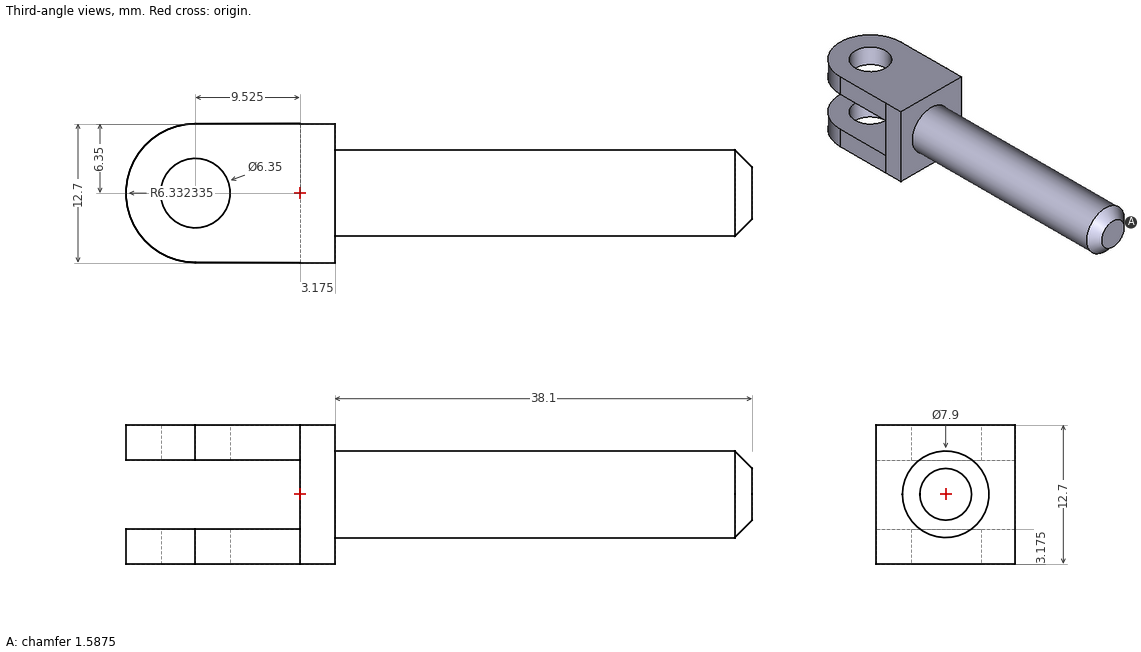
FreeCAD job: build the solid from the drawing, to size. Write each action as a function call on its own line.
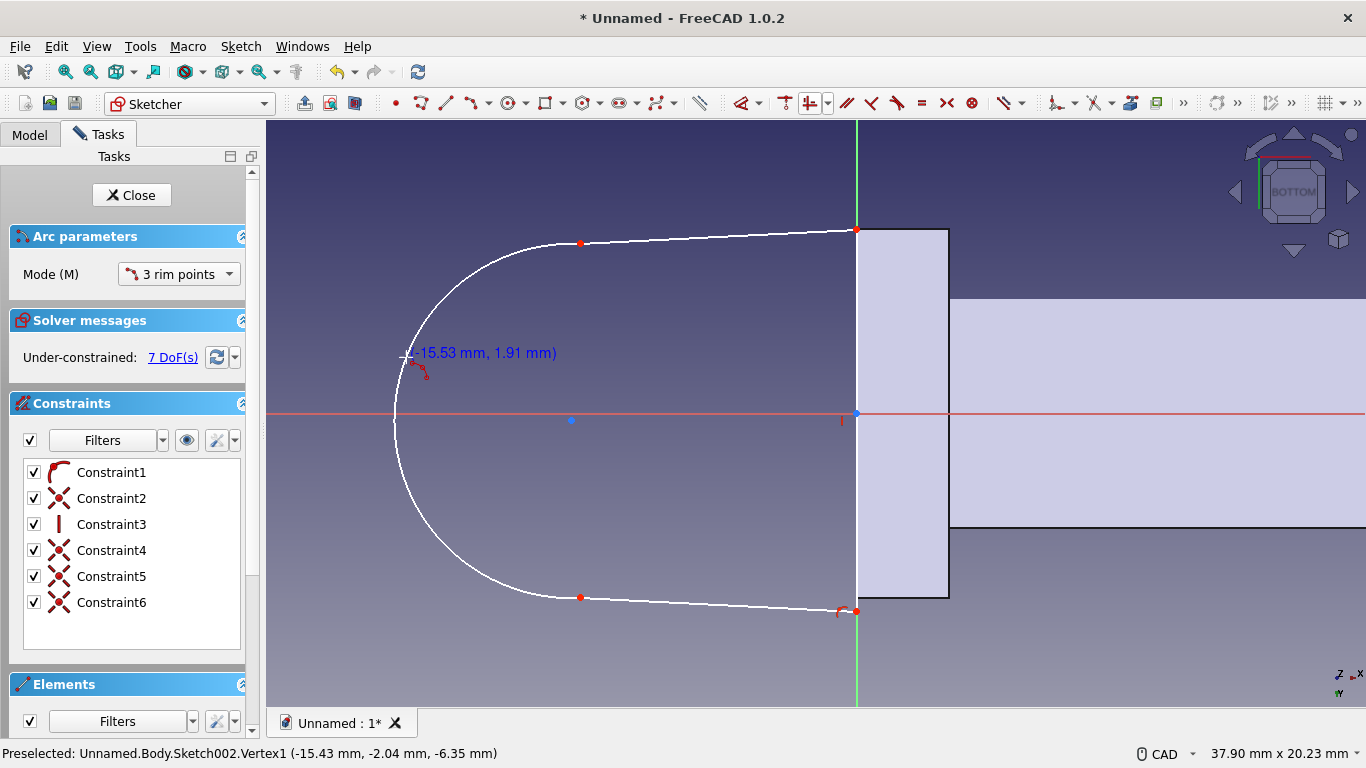
click(508, 104)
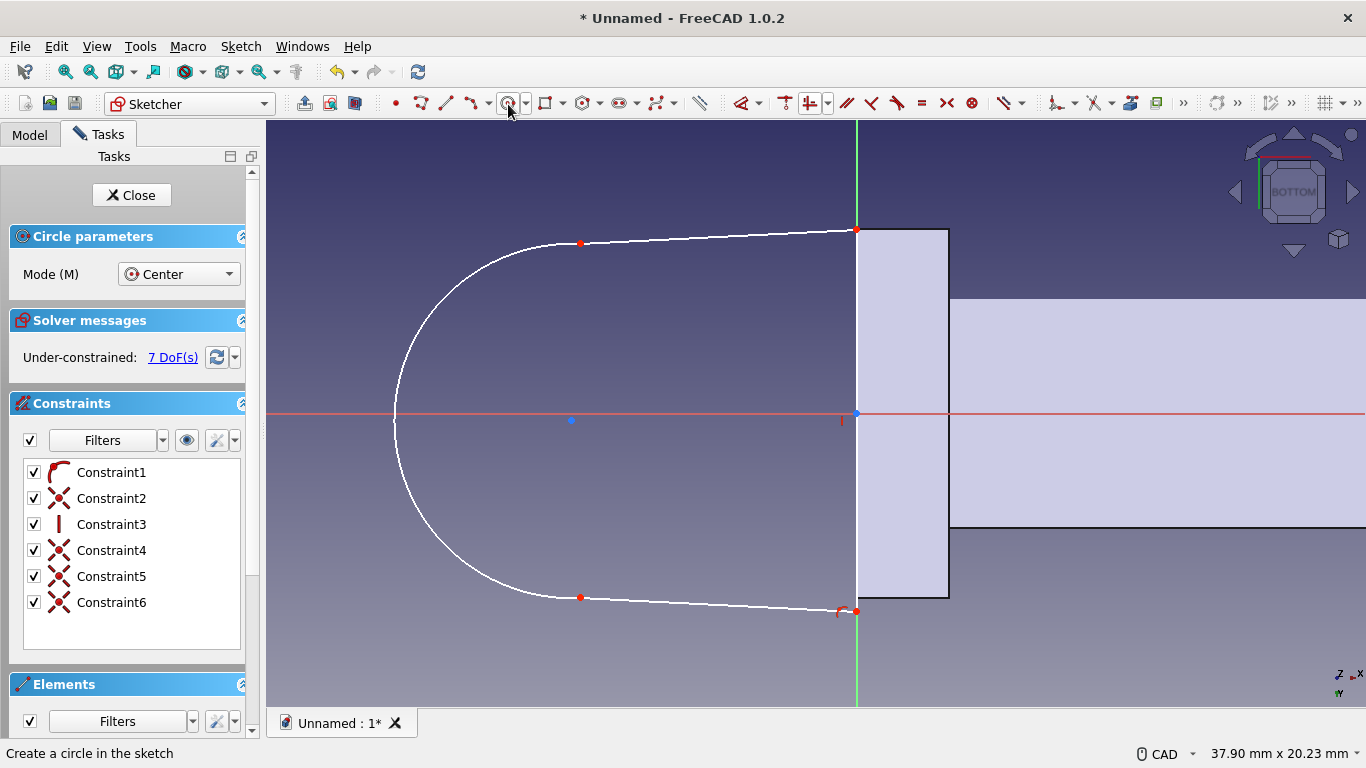
click(580, 414)
move(645, 348)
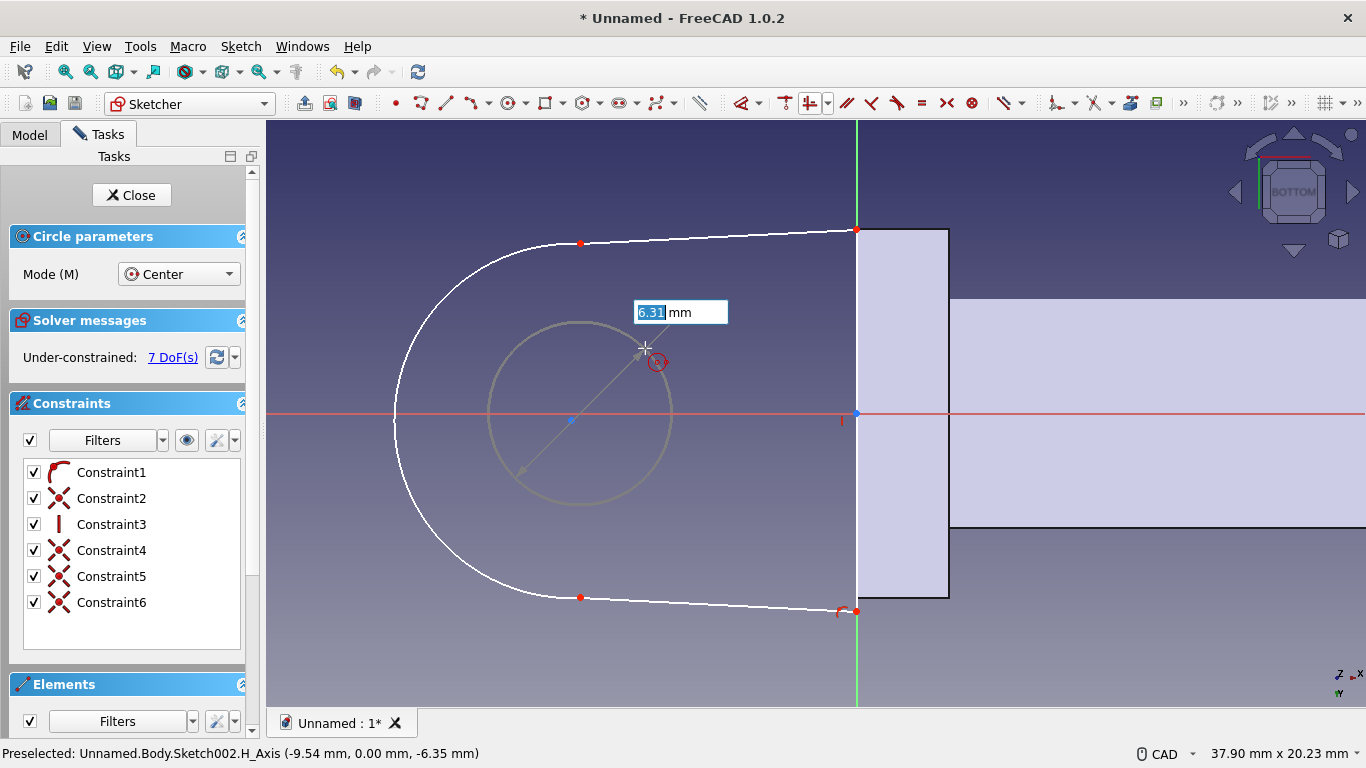
text(6.35)
key(Return)
key(Escape)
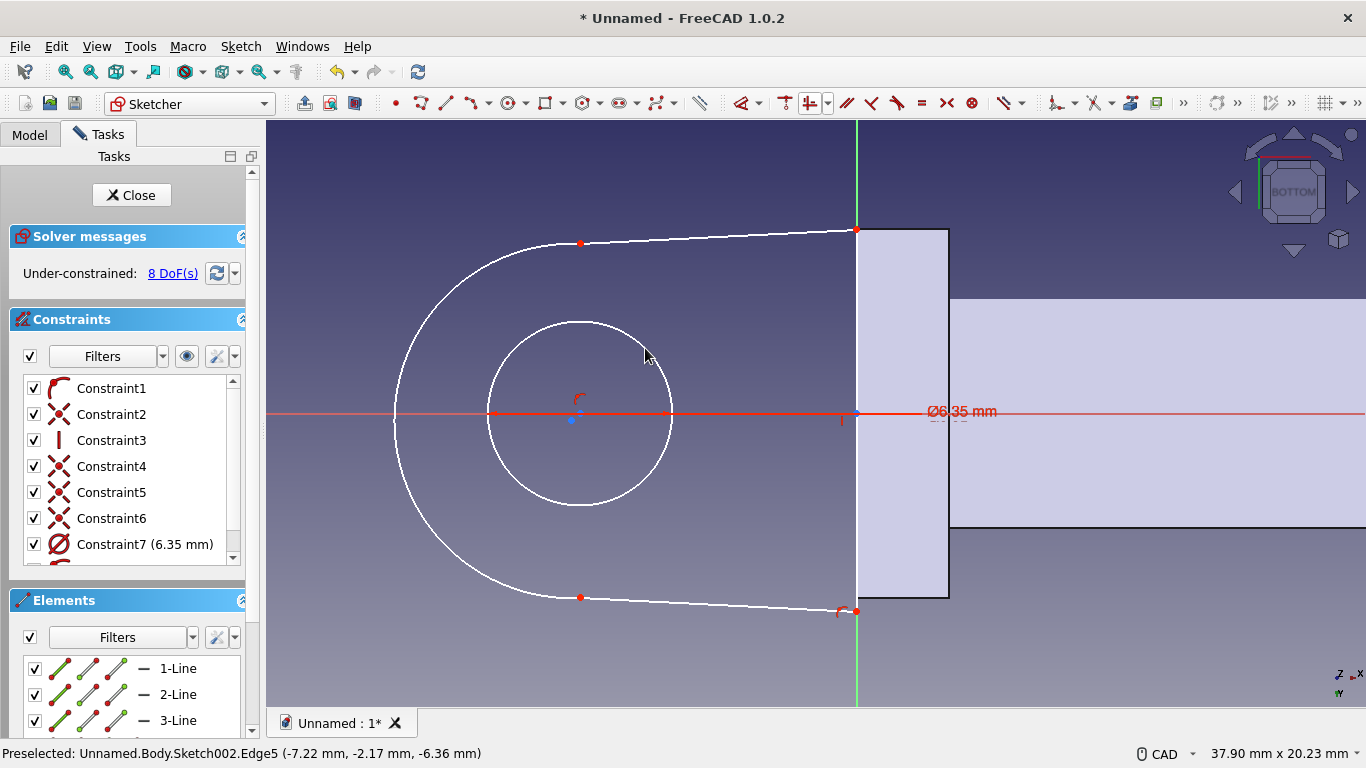
click(645, 348)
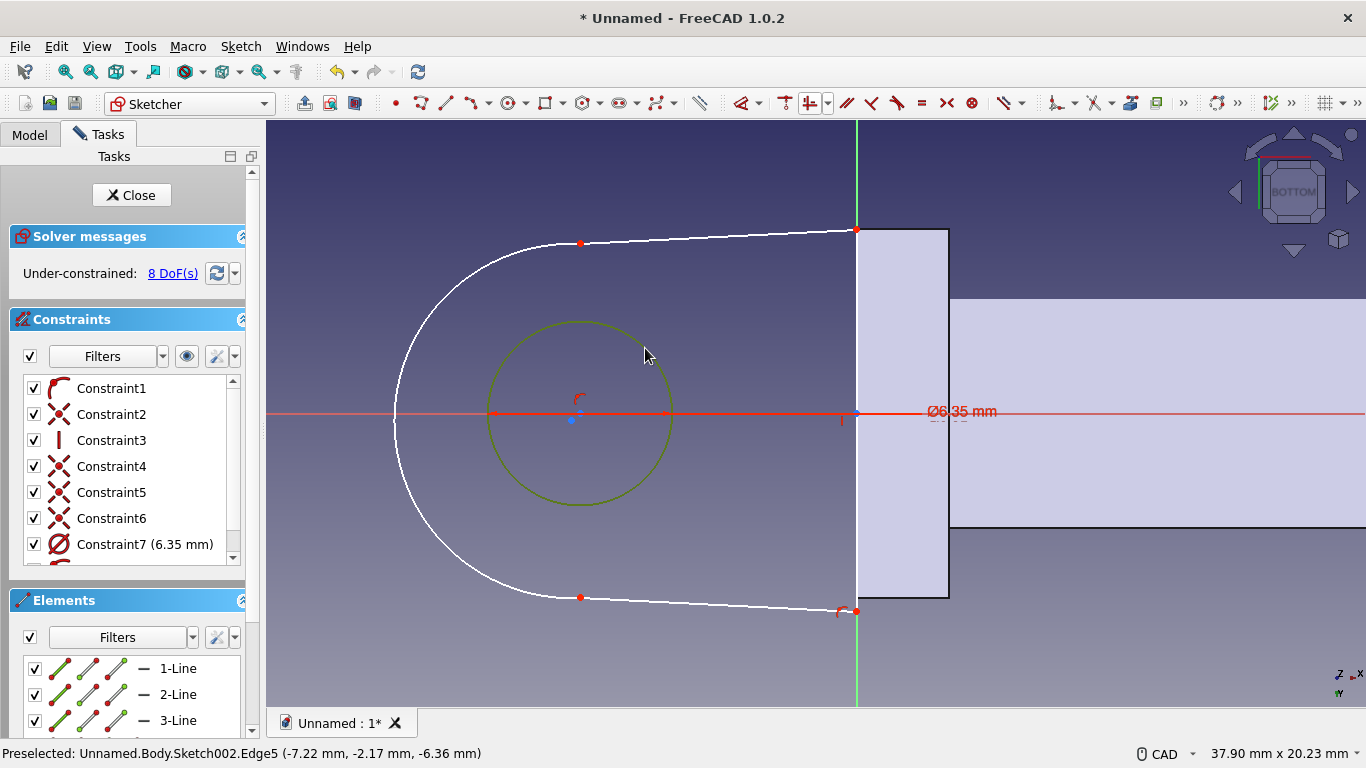
click(430, 314)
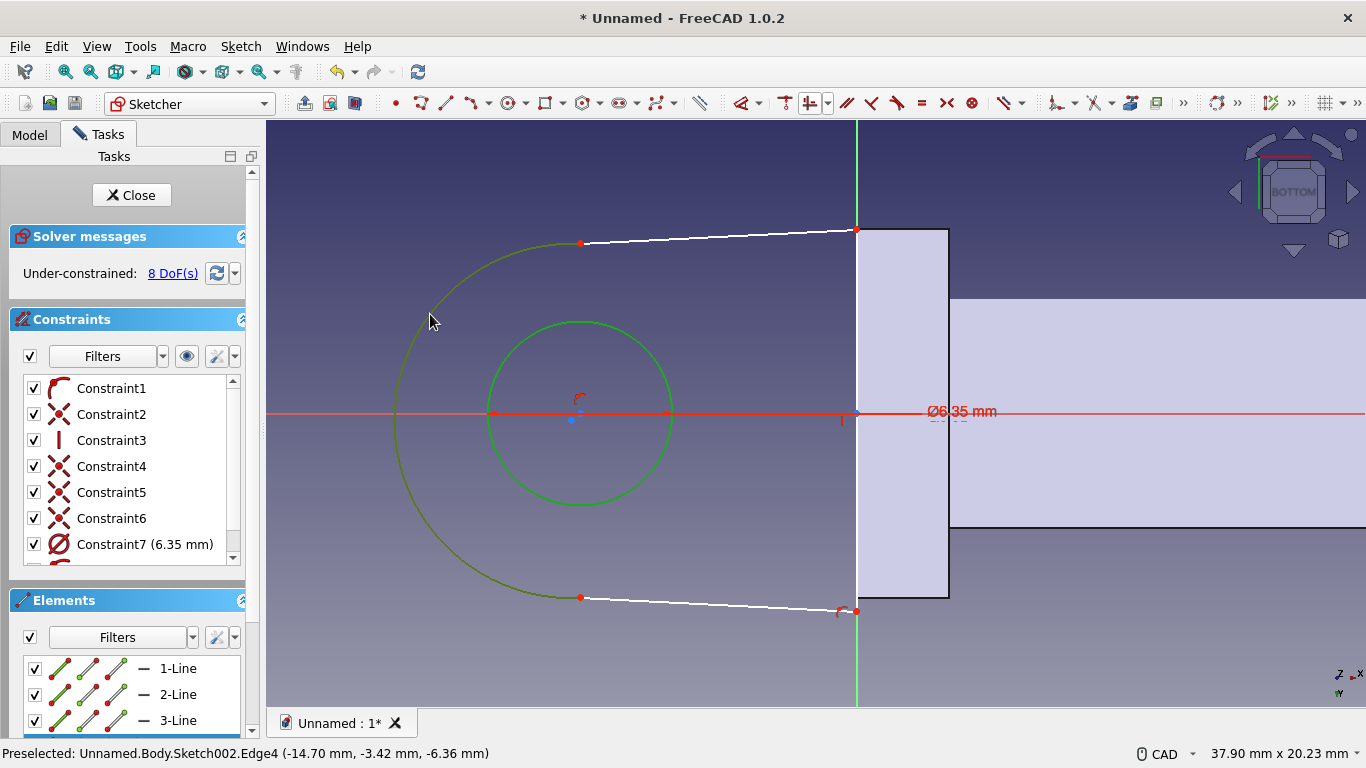
click(785, 104)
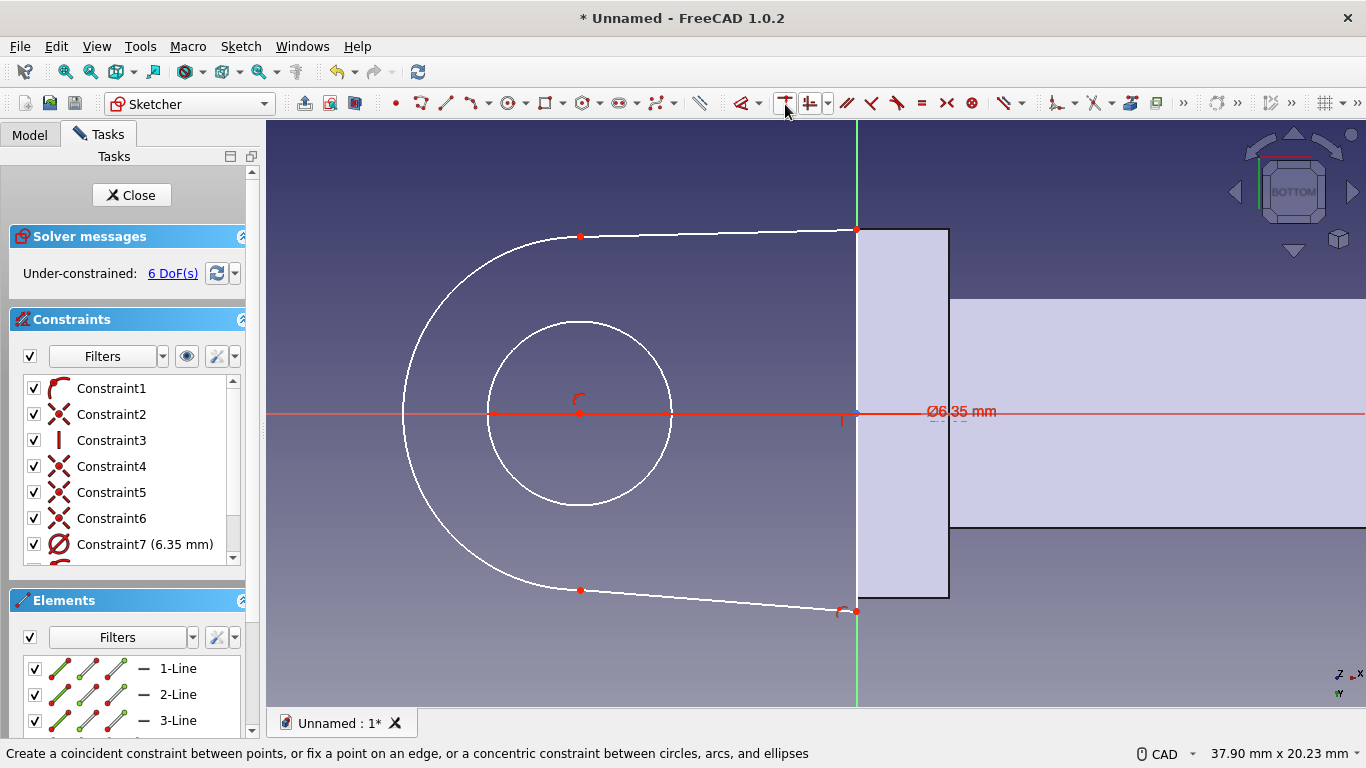
click(740, 104)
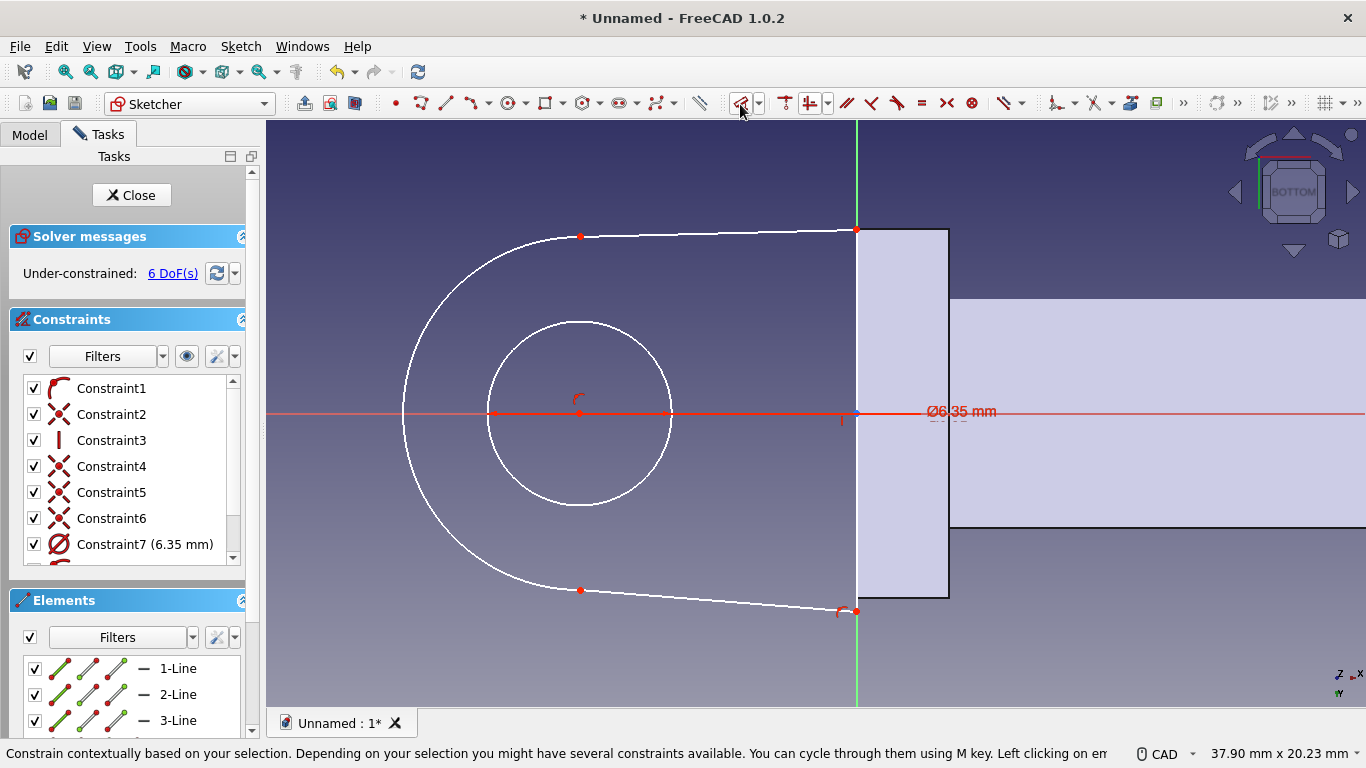
click(437, 310)
click(411, 291)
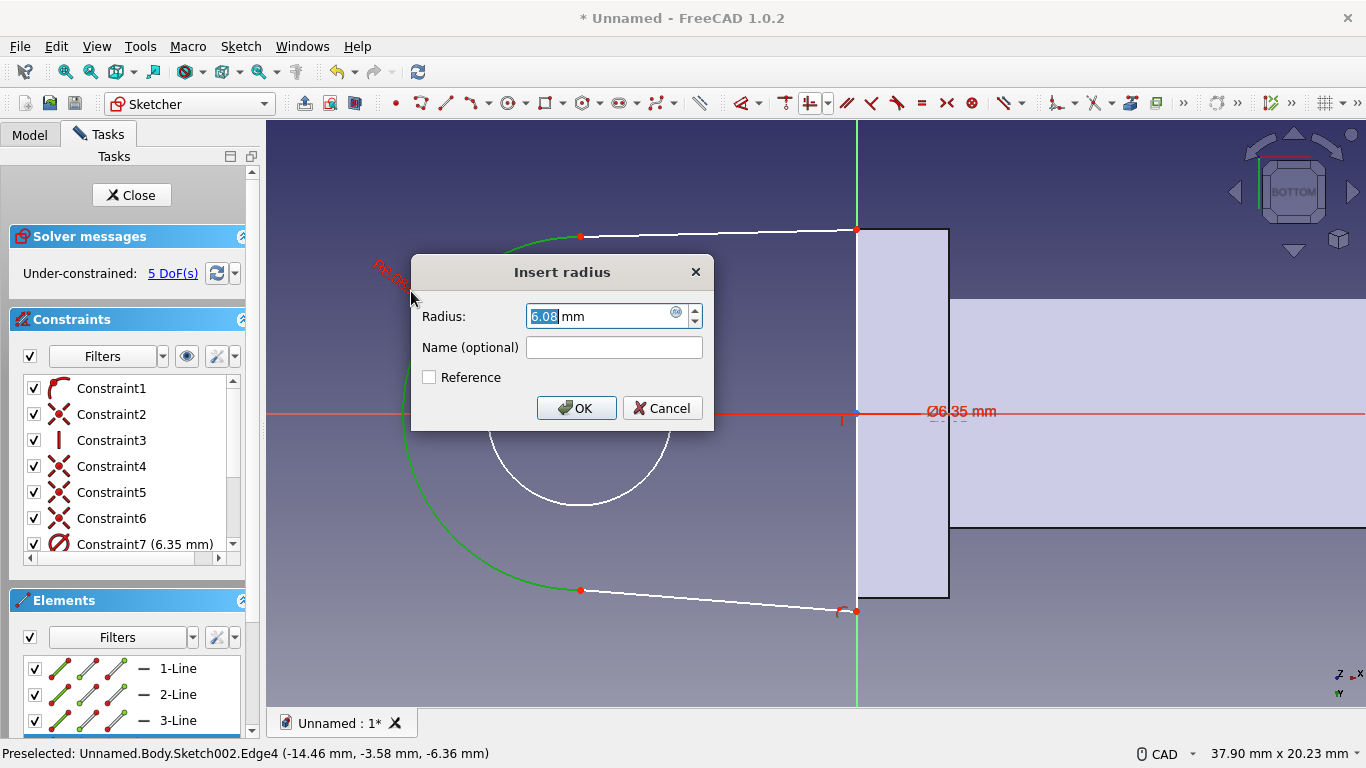
text(6.332335)
key(Return)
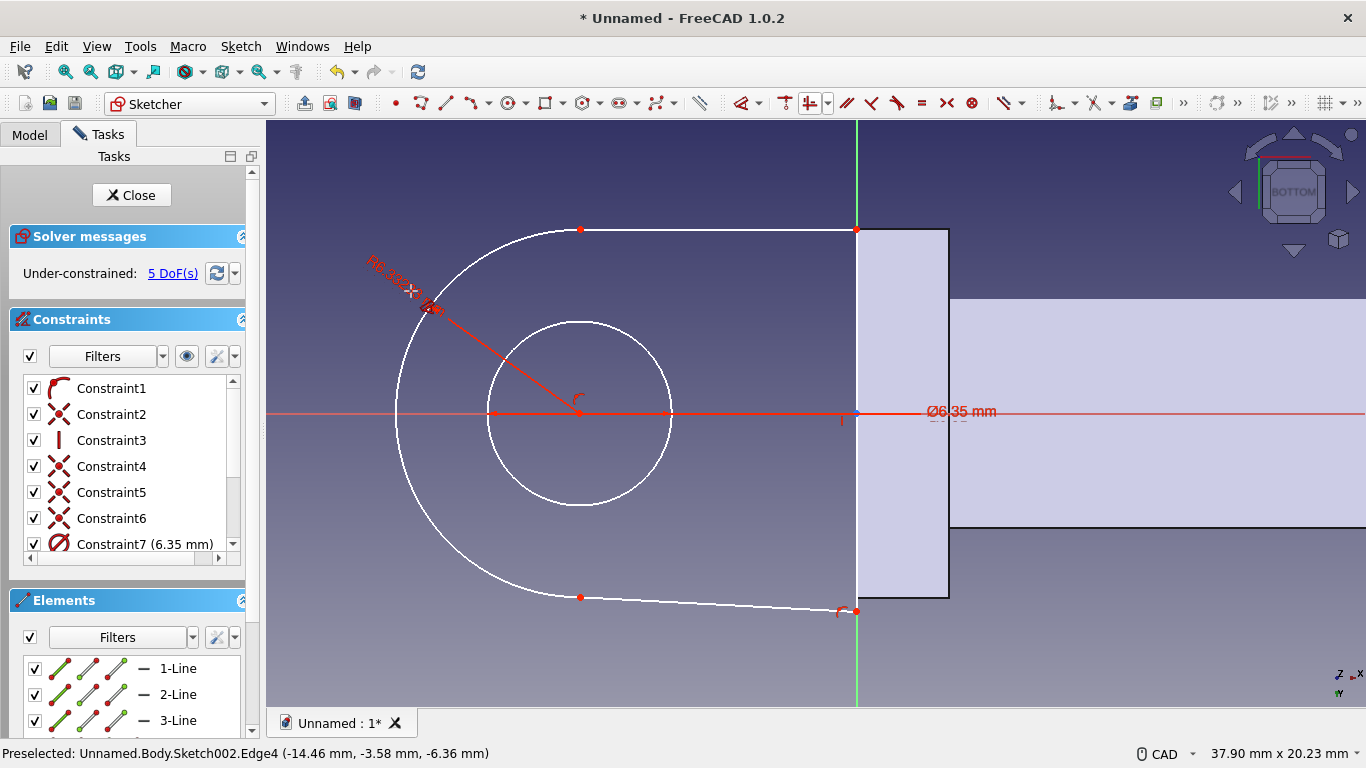
click(857, 497)
click(891, 333)